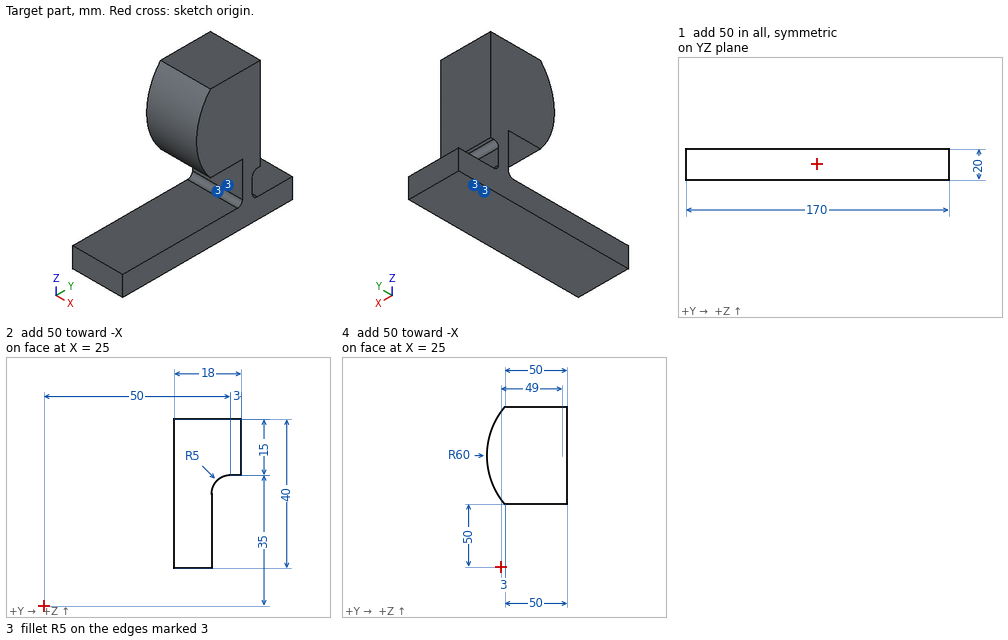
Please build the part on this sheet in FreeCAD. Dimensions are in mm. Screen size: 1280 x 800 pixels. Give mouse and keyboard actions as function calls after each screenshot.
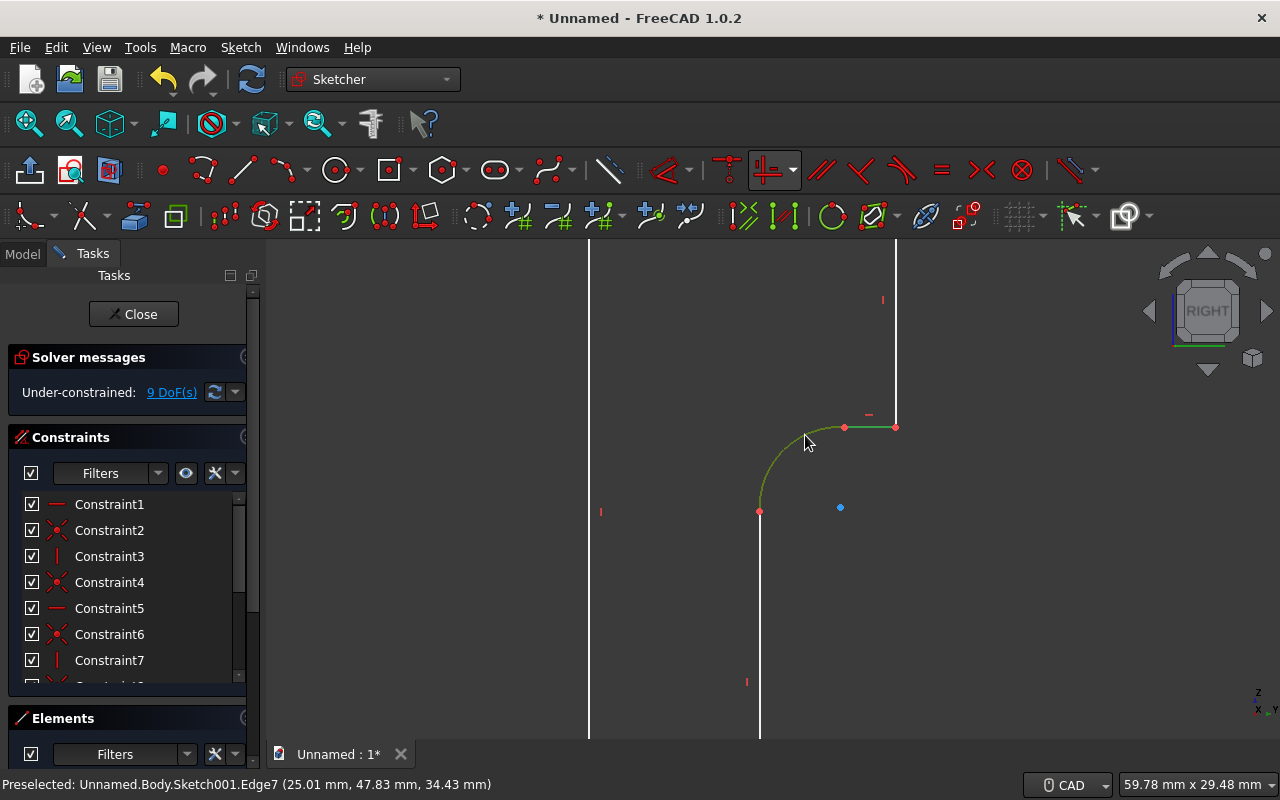
key(t)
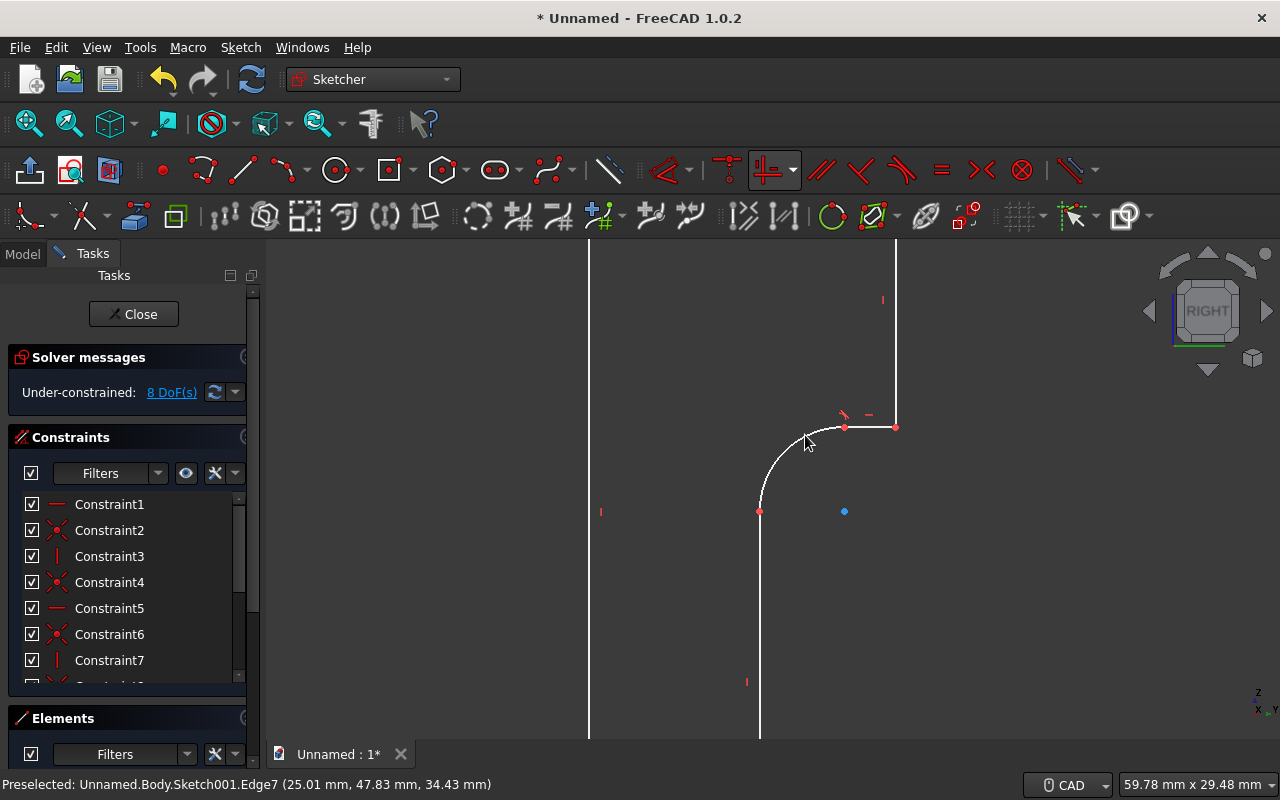
click(760, 613)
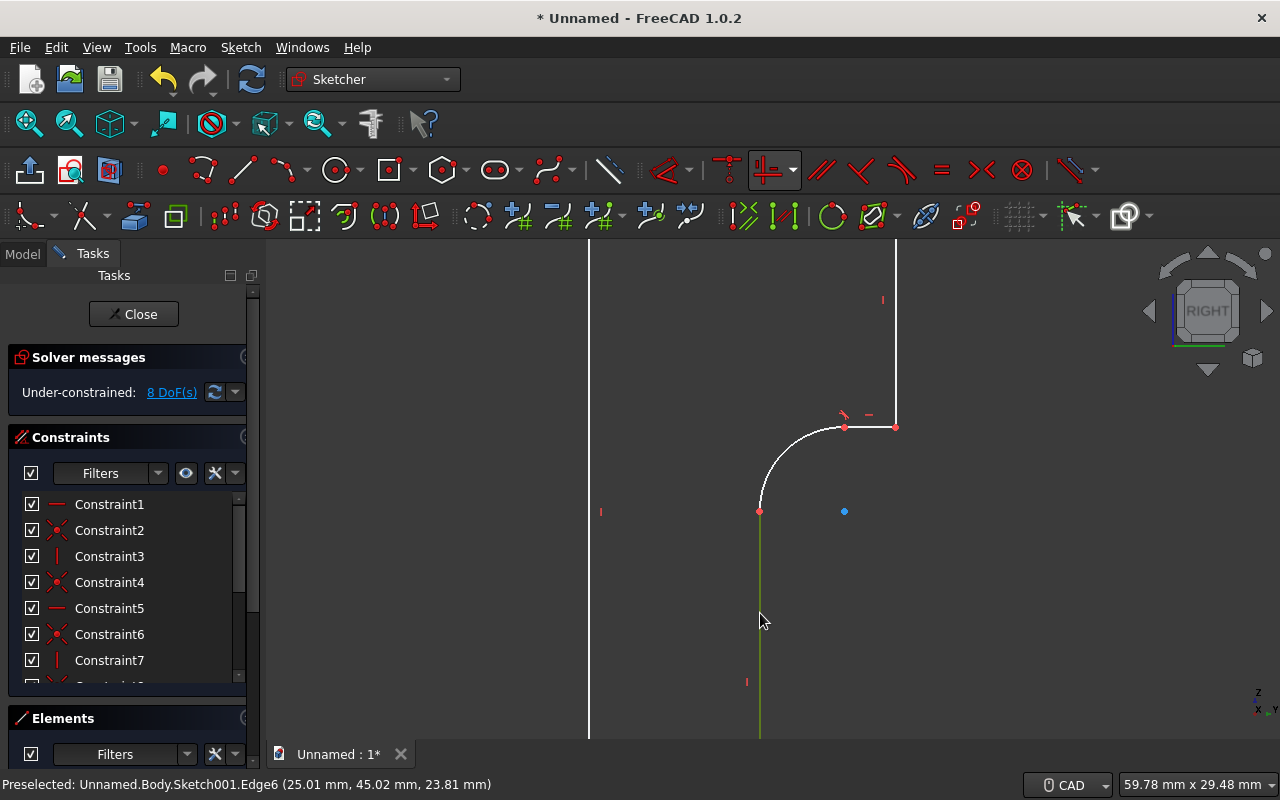
click(806, 436)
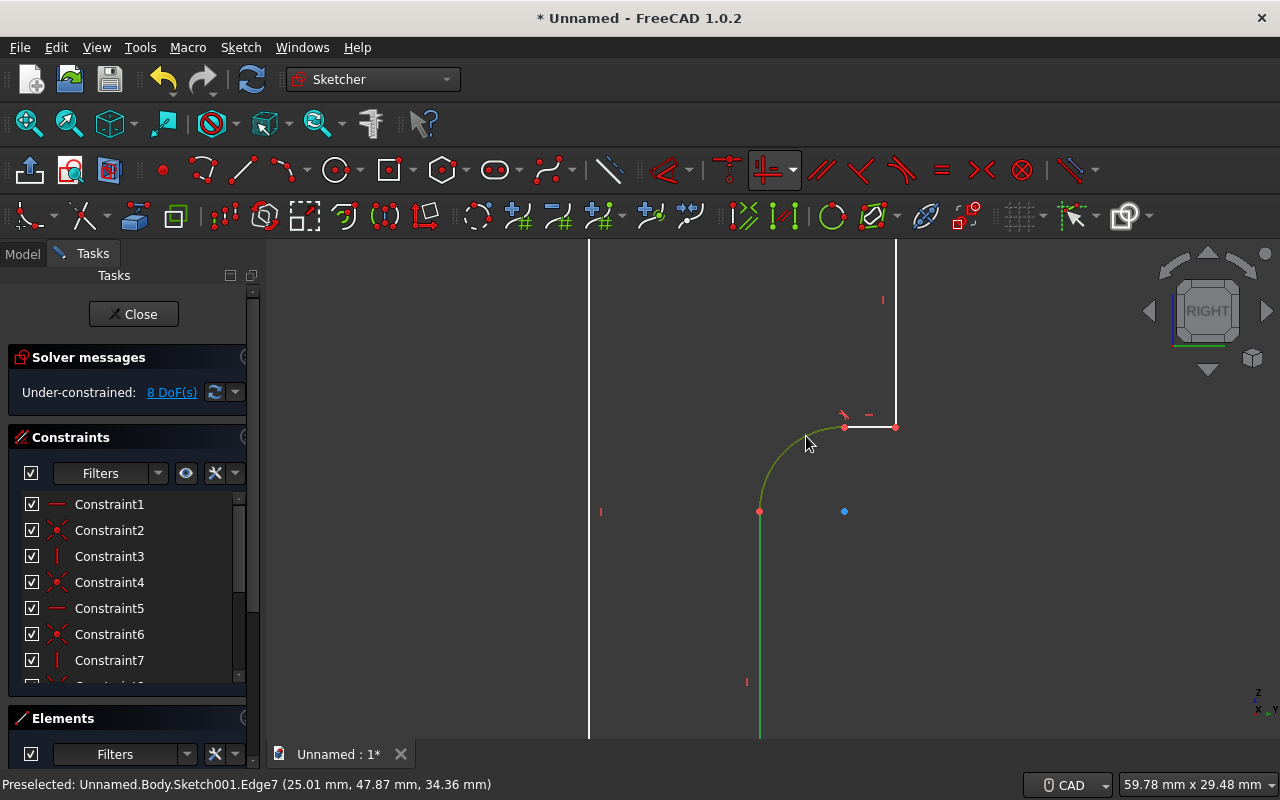
key(t)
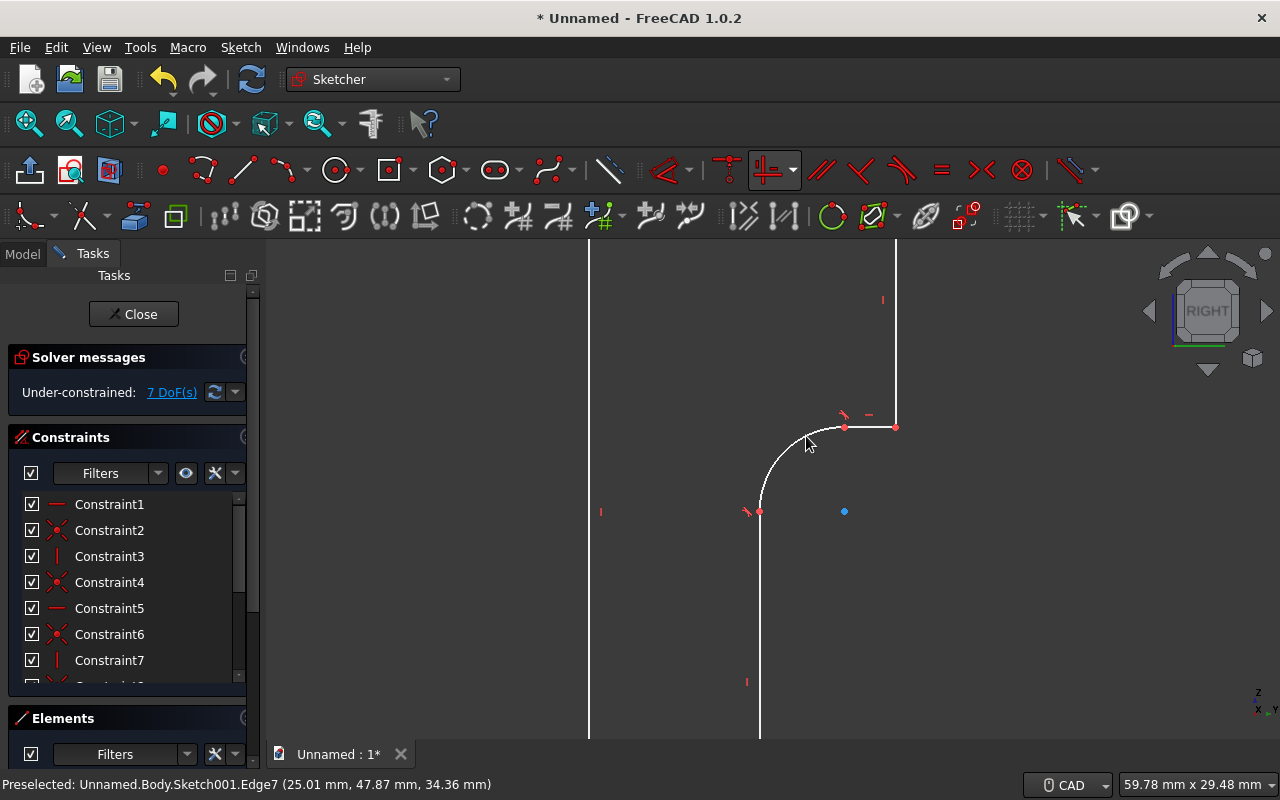
click(664, 170)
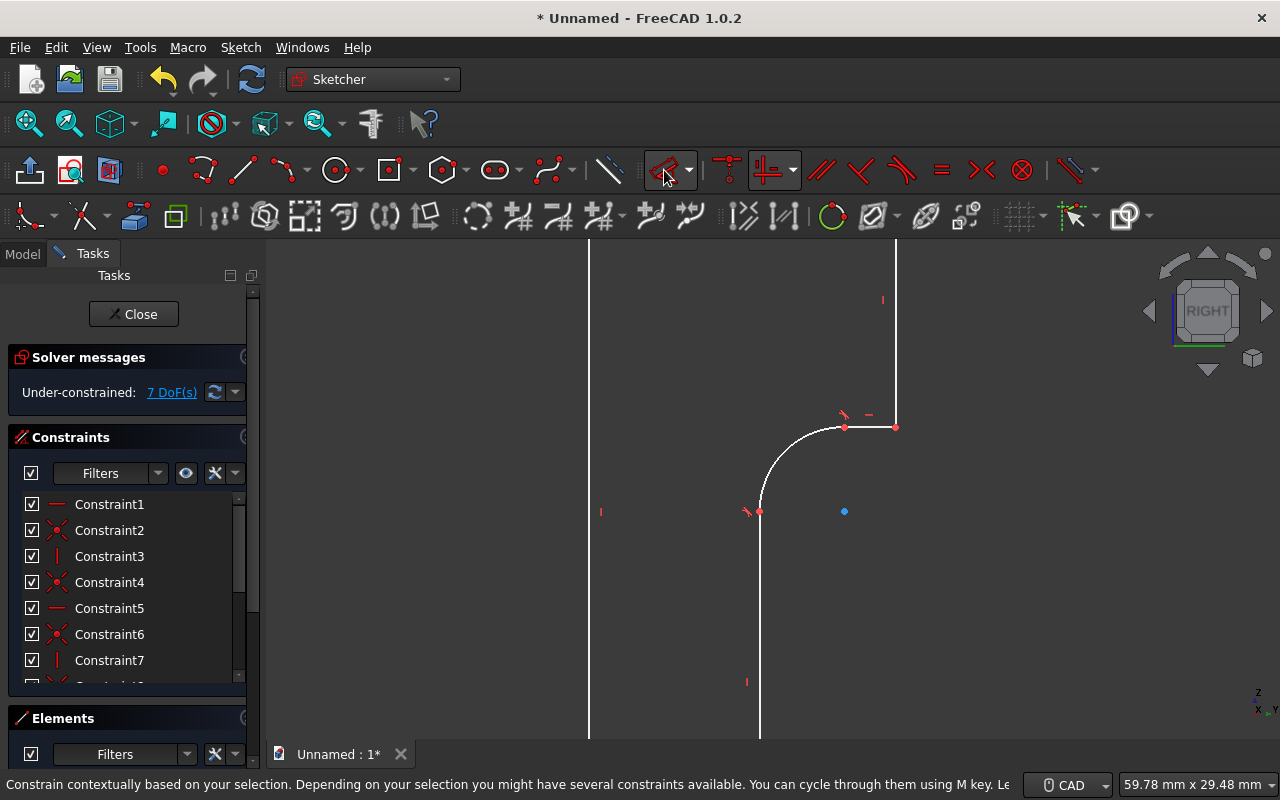
click(806, 436)
click(792, 407)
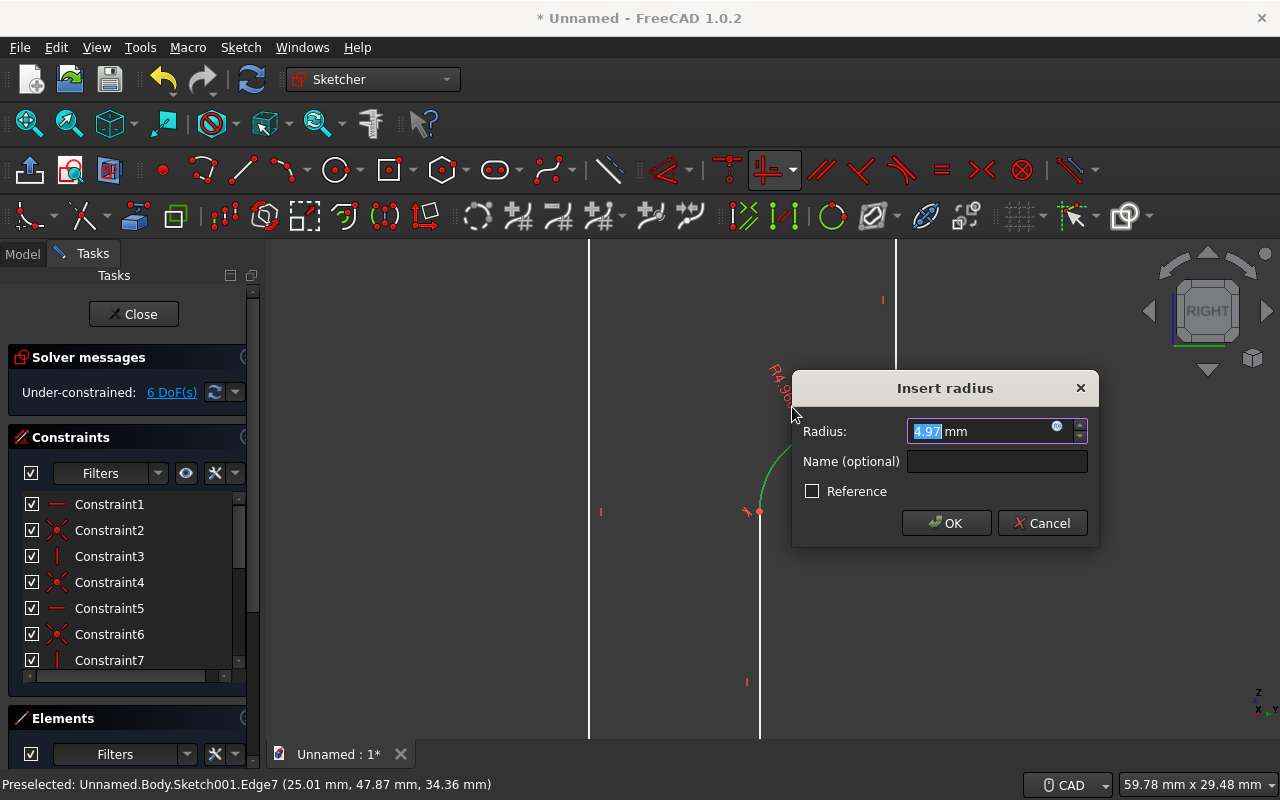
text(5)
key(Return)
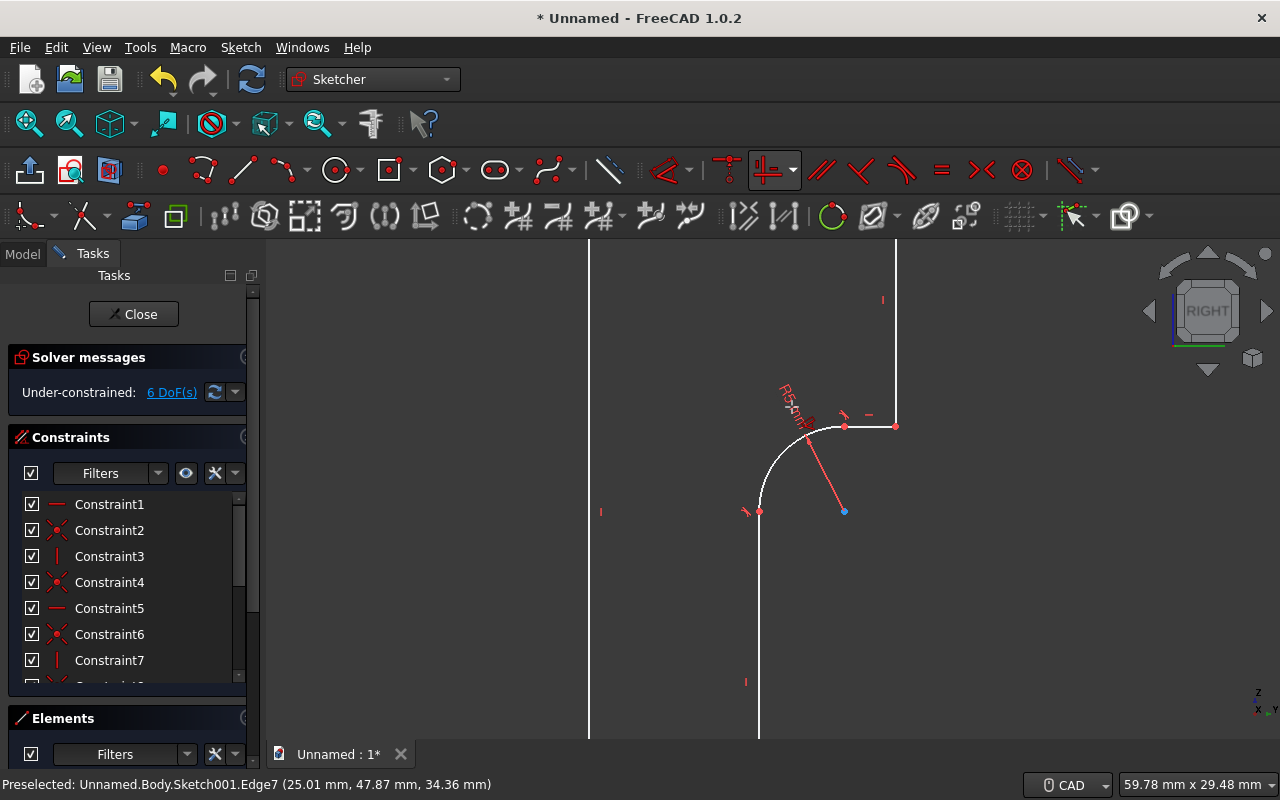
click(860, 427)
click(870, 393)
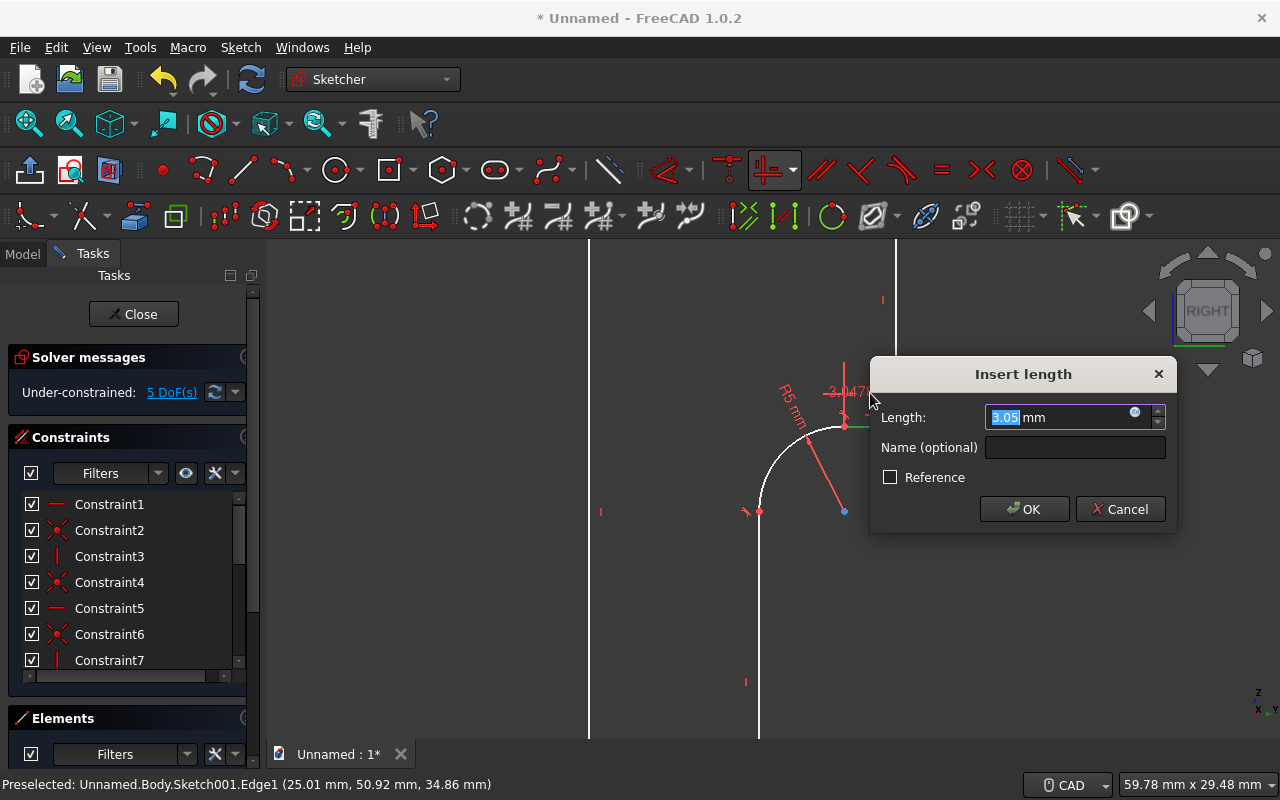
text(3)
key(Return)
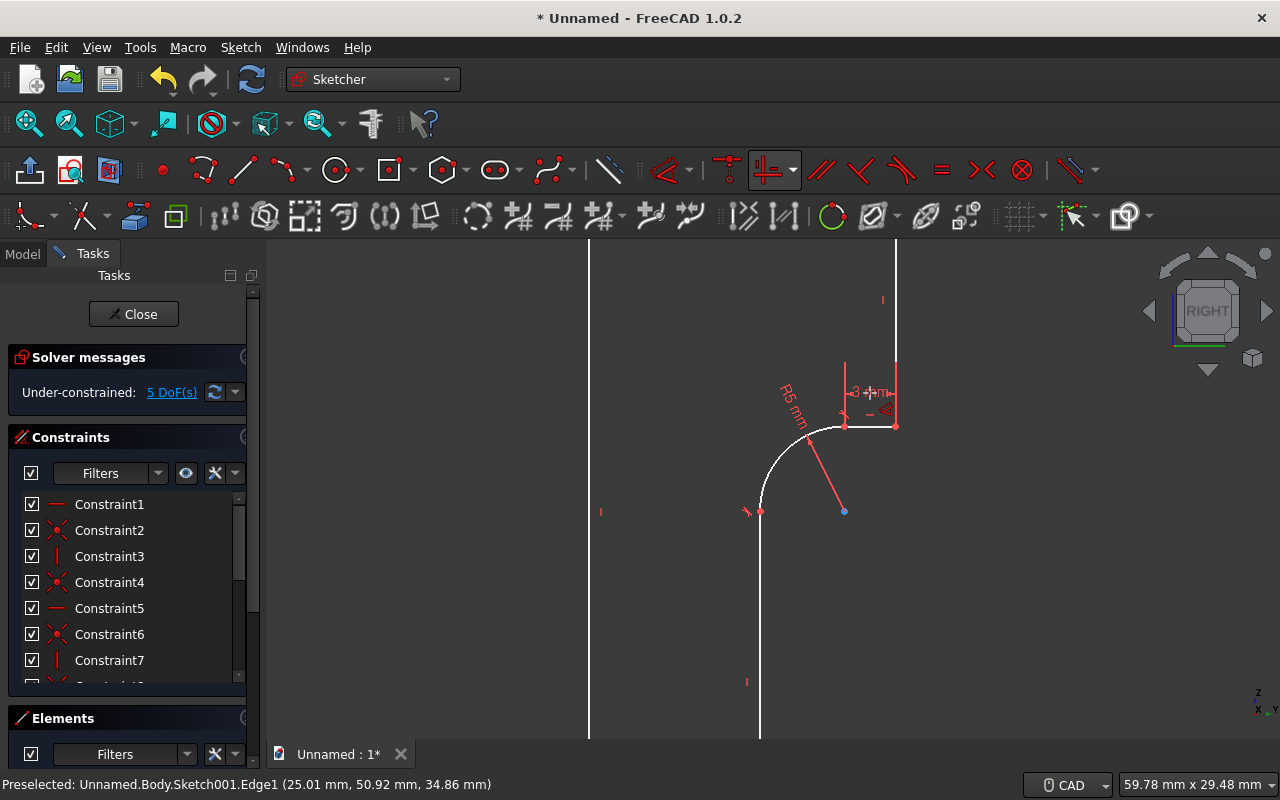
click(896, 350)
click(930, 347)